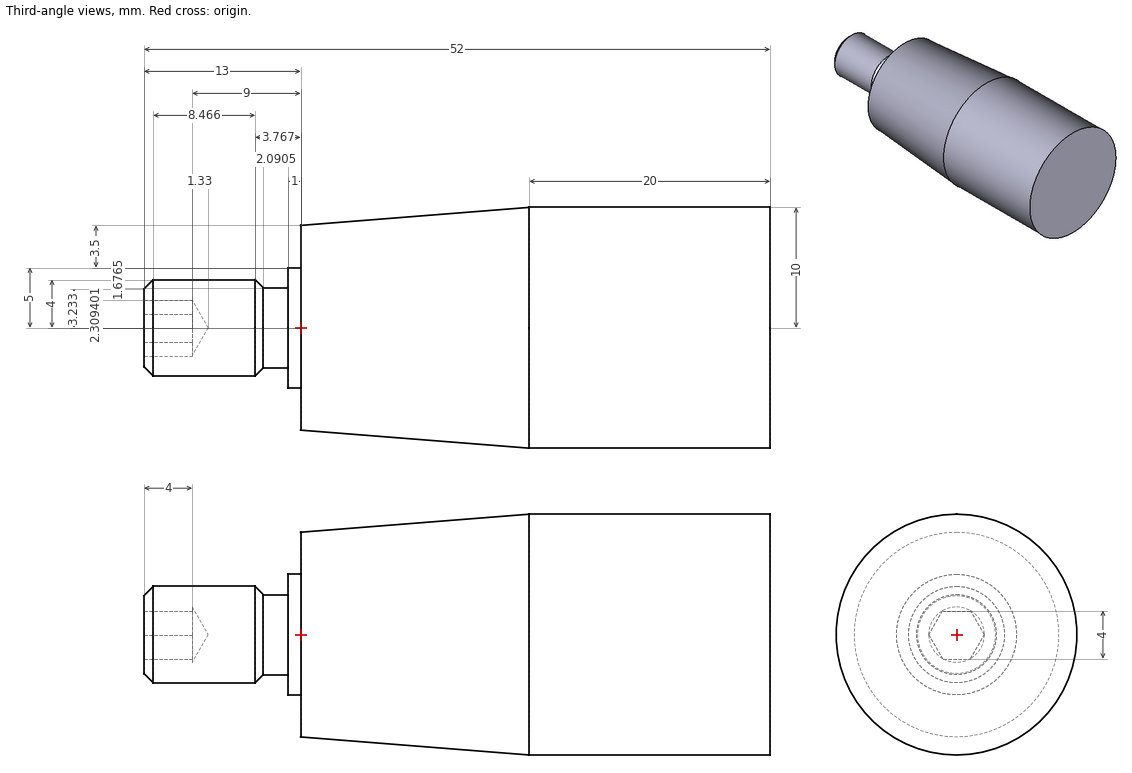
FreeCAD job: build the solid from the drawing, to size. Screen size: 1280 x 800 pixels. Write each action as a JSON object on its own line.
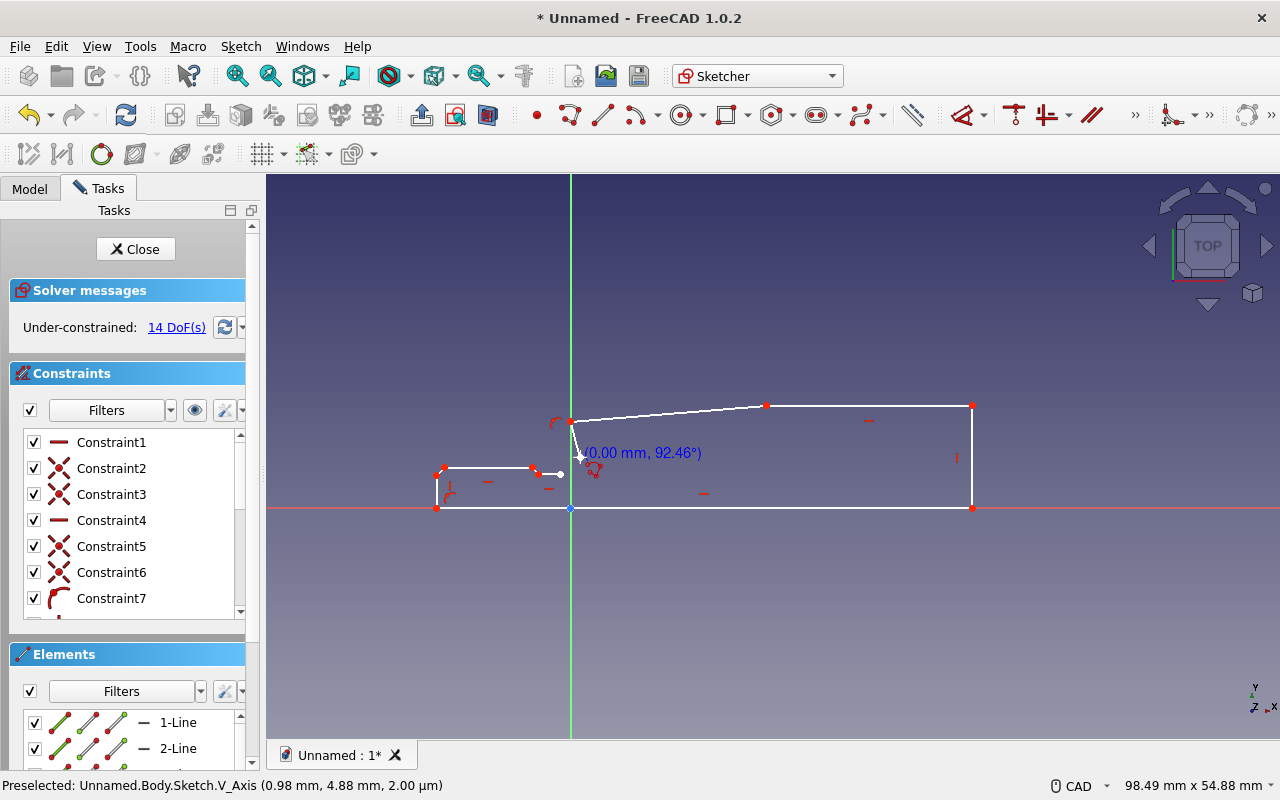
{"action": "scroll", "coordinate": [560, 457], "scroll_direction": "up", "scroll_amount": 3}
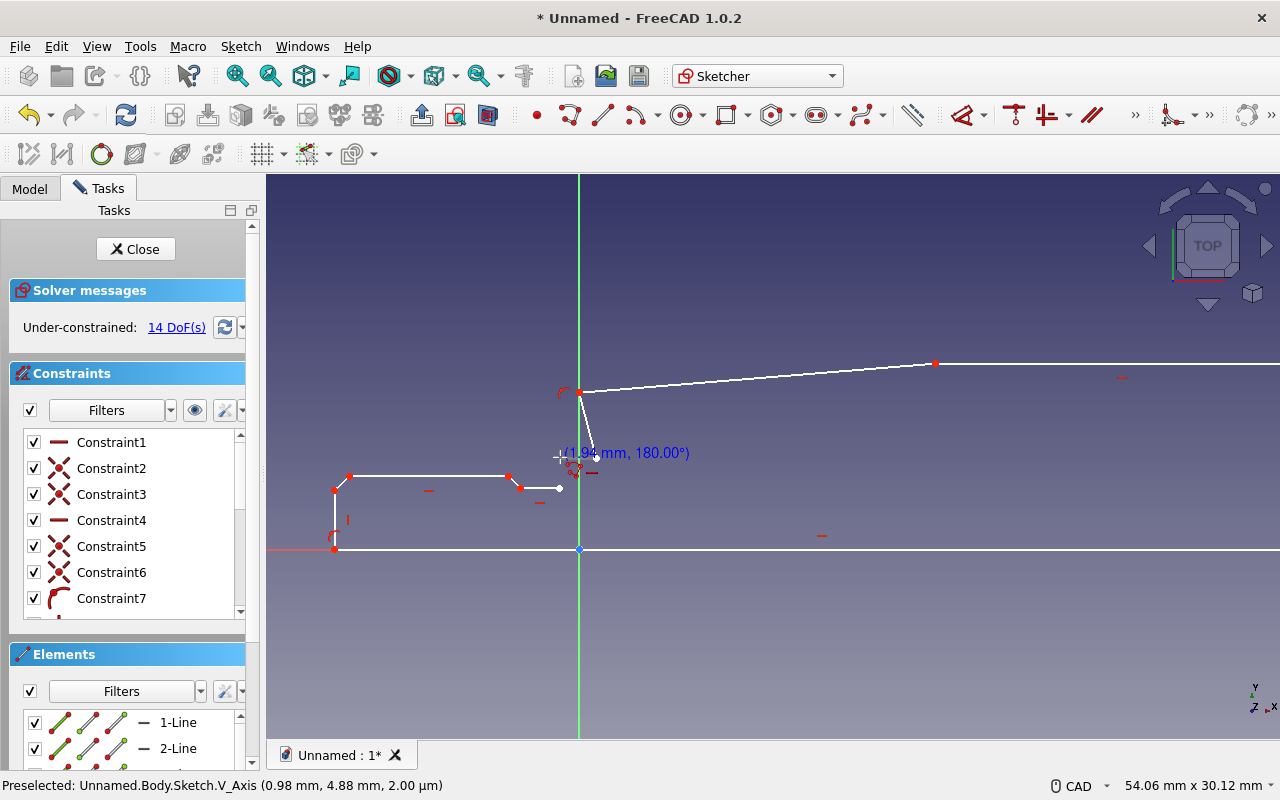
{"action": "left_click", "coordinate": [560, 457]}
{"action": "left_click", "coordinate": [560, 488]}
{"action": "key", "text": "Escape"}
{"action": "key", "text": "Escape"}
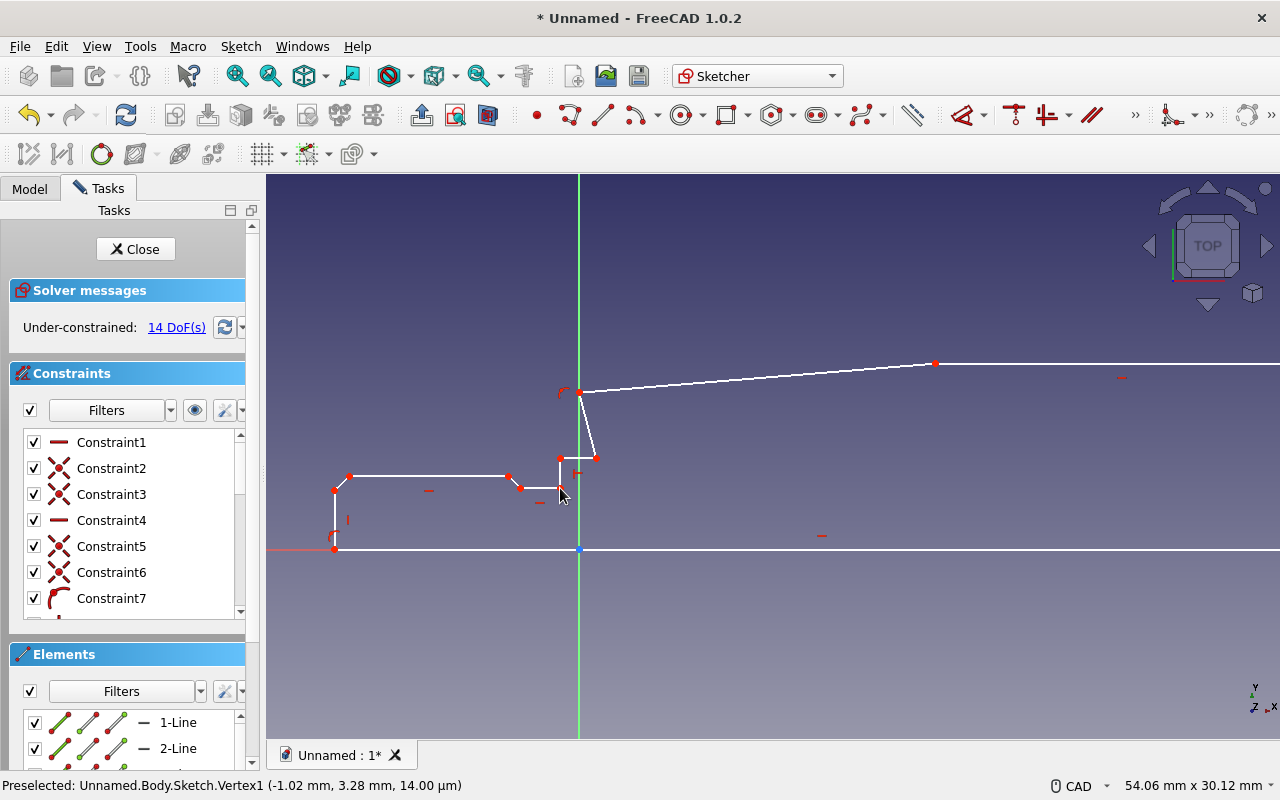
{"action": "left_click", "coordinate": [591, 439]}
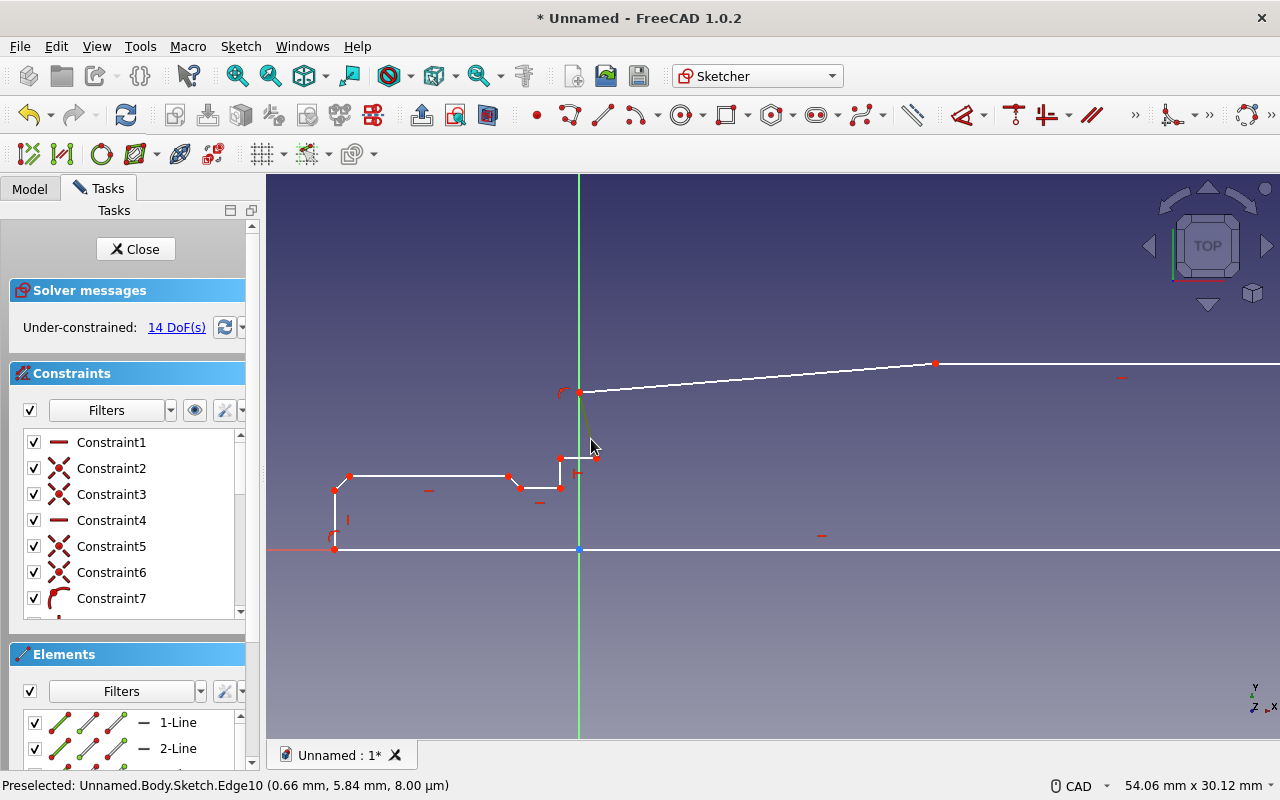
{"action": "key", "text": "v"}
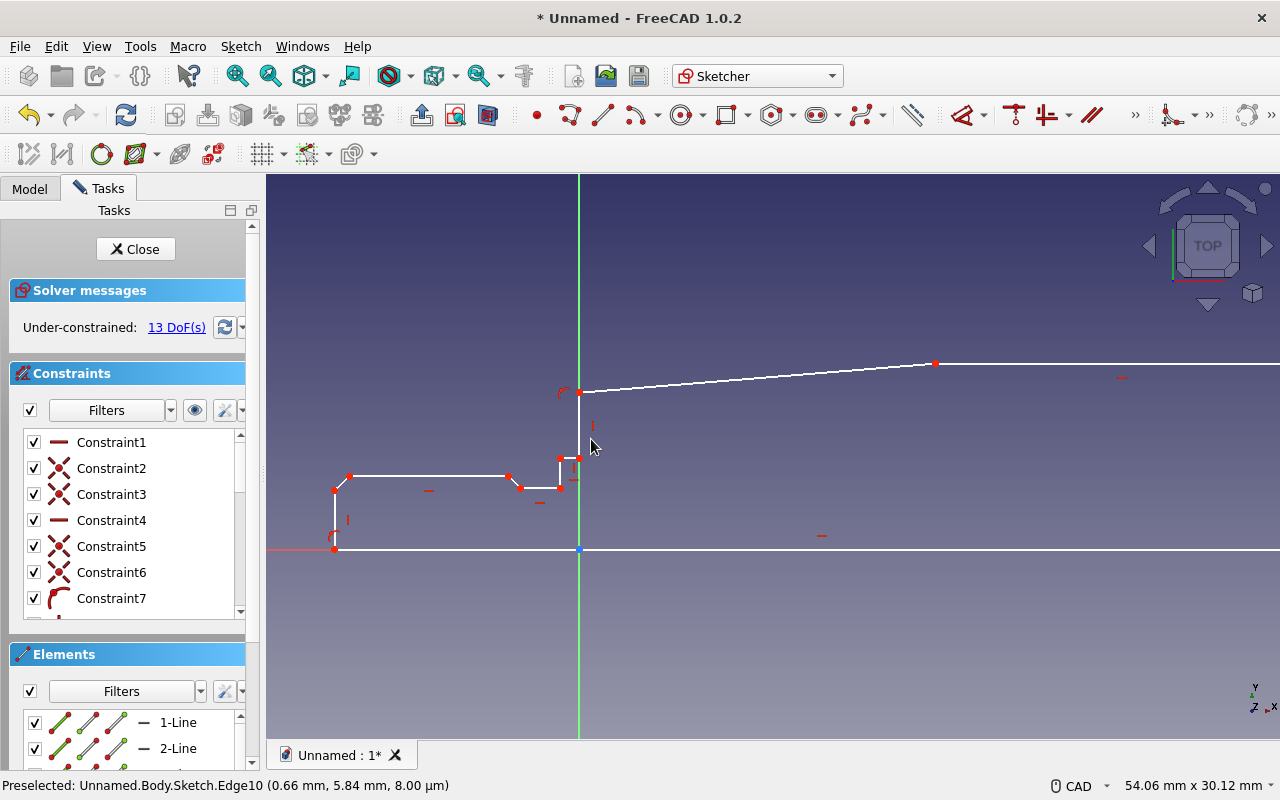
{"action": "left_click", "coordinate": [962, 116]}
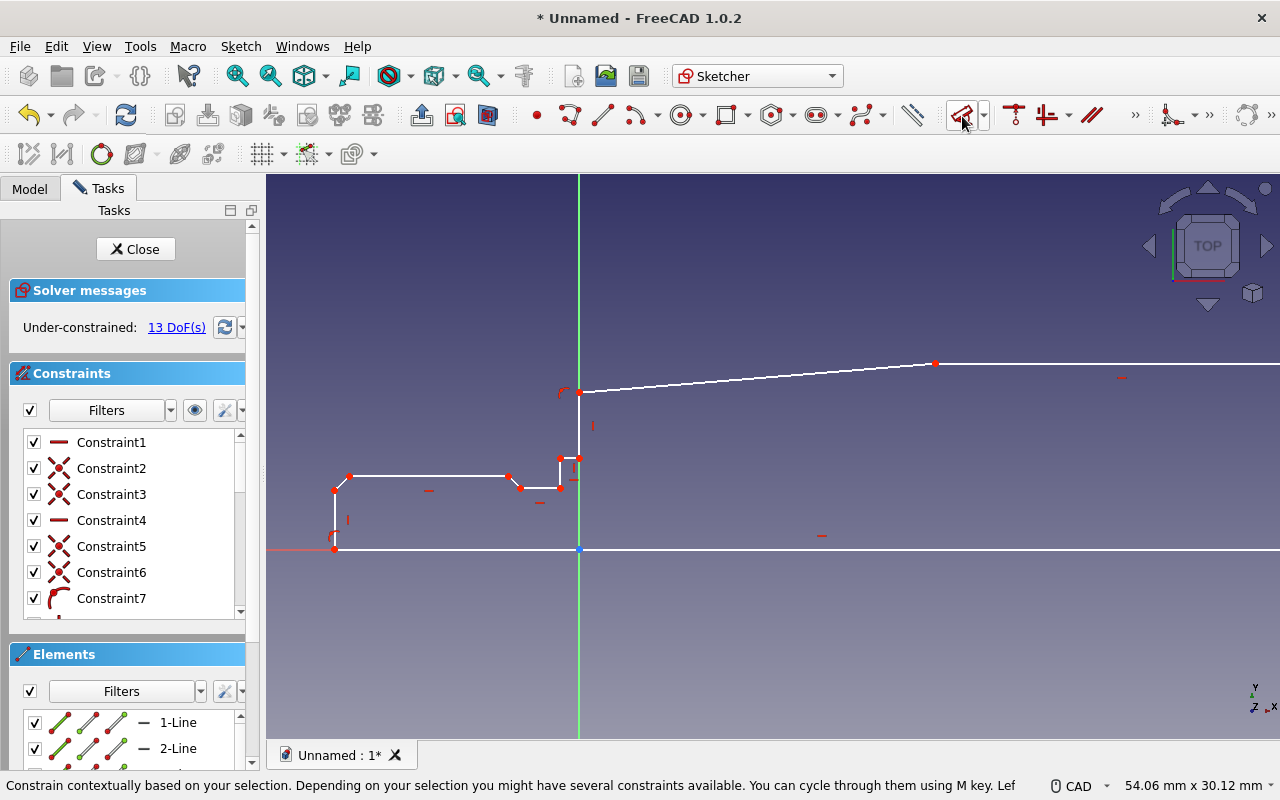
{"action": "scroll", "coordinate": [570, 458], "scroll_direction": "up", "scroll_amount": 4}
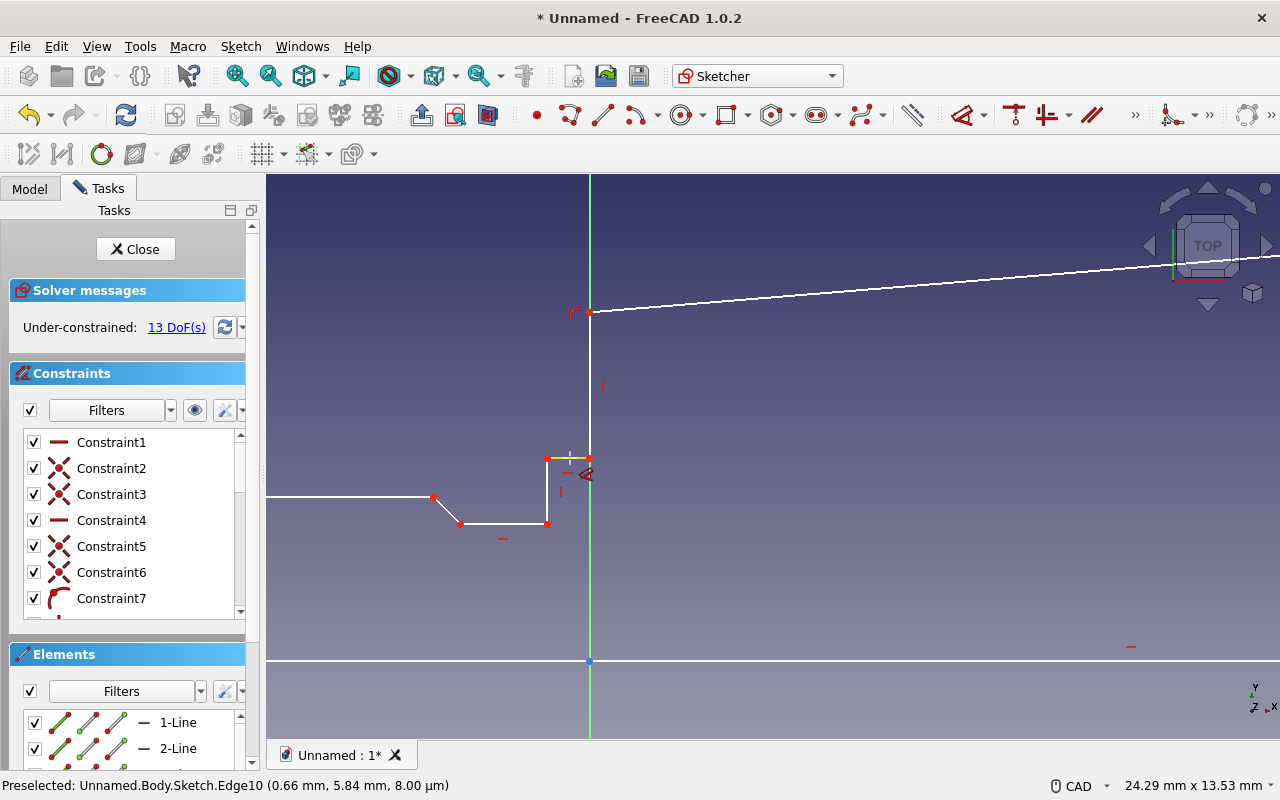
{"action": "left_click", "coordinate": [569, 458]}
{"action": "left_click", "coordinate": [569, 492]}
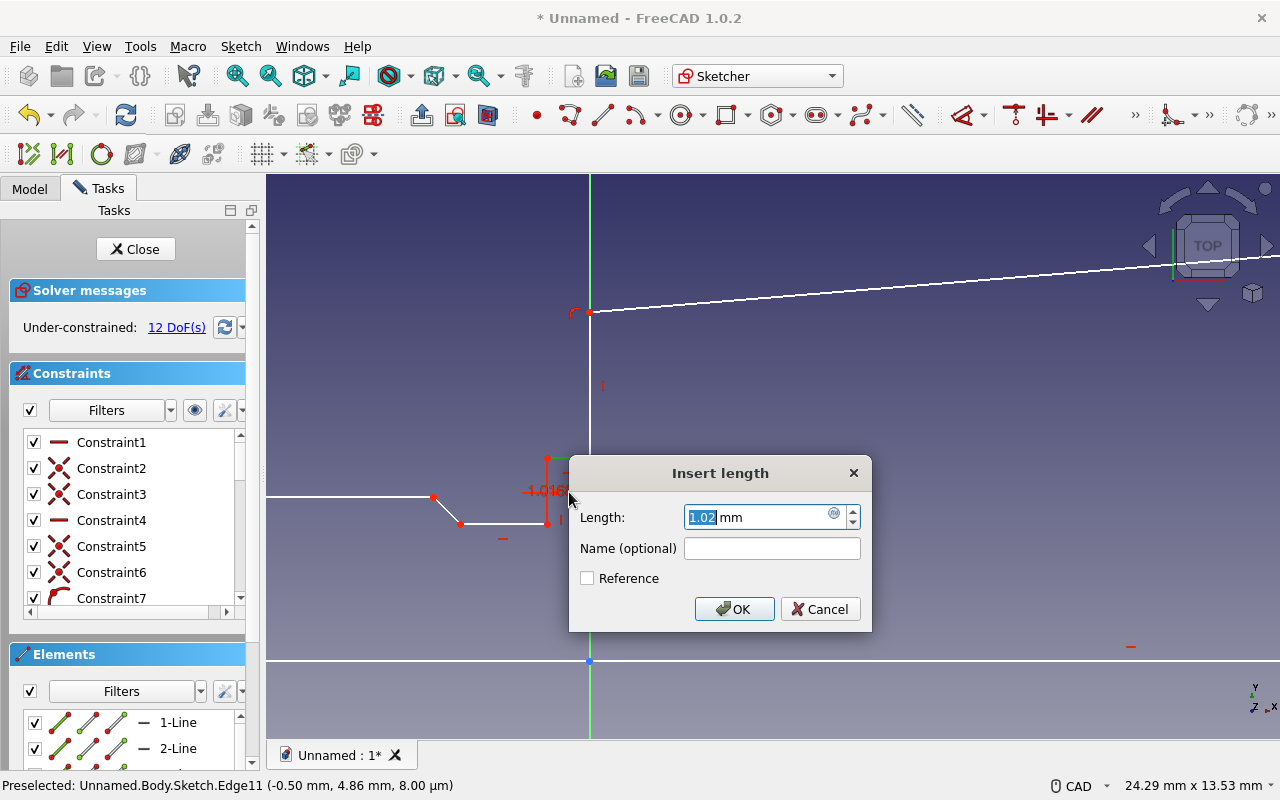
{"action": "type", "text": "1"}
{"action": "key", "text": "Return"}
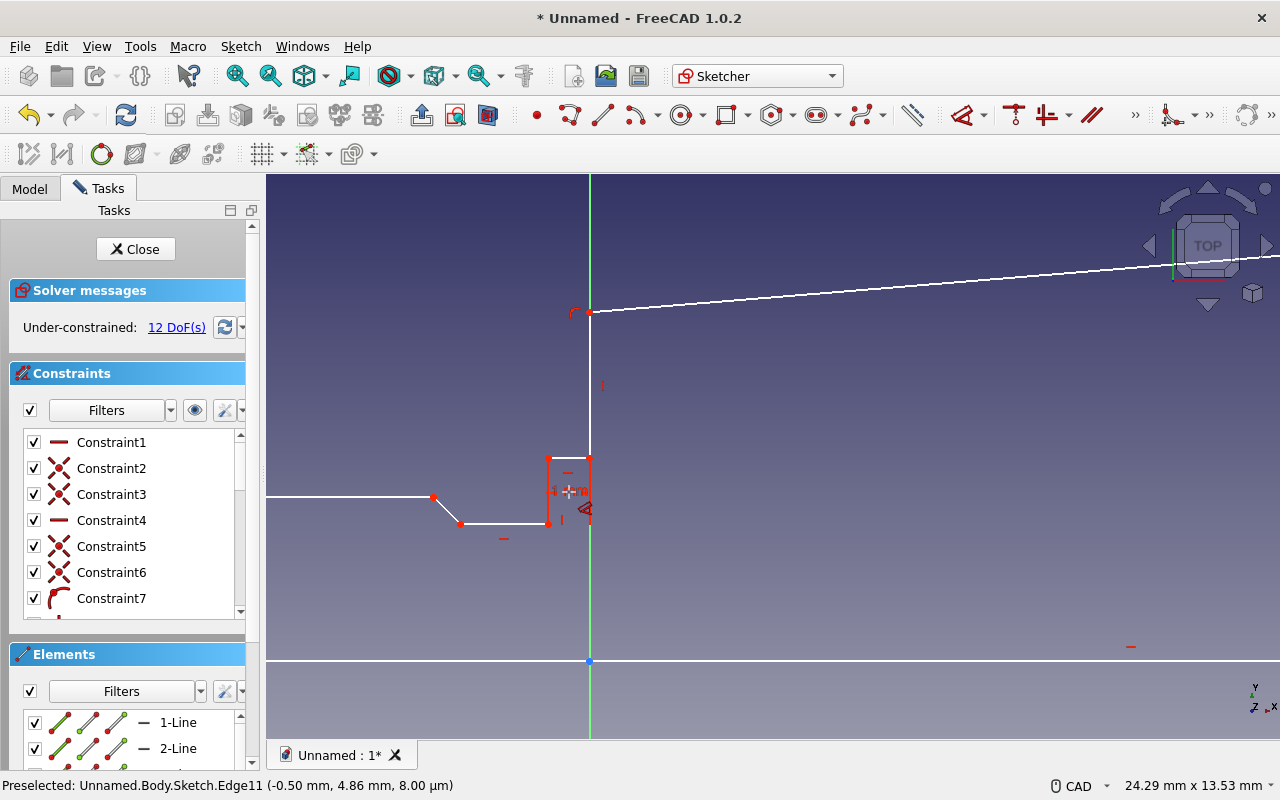
{"action": "scroll", "coordinate": [564, 458], "scroll_direction": "down", "scroll_amount": 7}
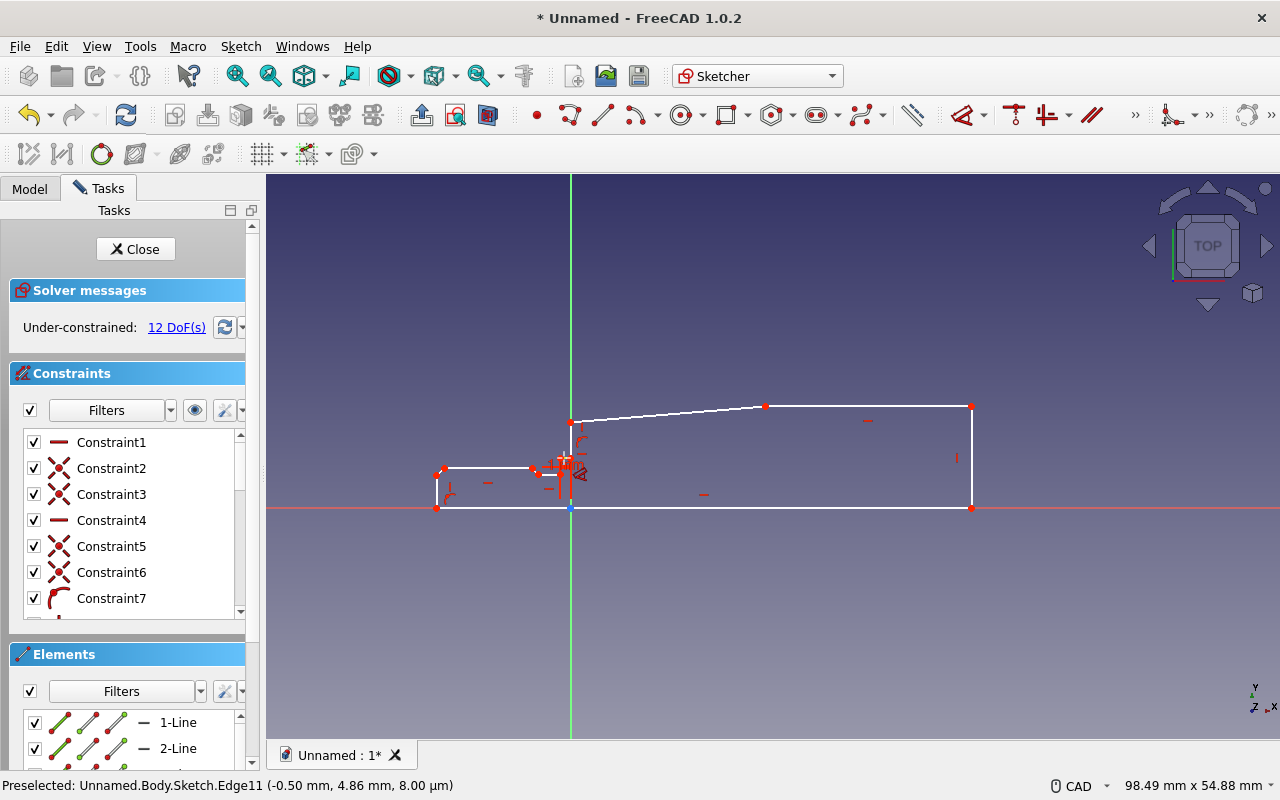
{"action": "left_click", "coordinate": [597, 508]}
{"action": "left_click", "coordinate": [704, 542]}